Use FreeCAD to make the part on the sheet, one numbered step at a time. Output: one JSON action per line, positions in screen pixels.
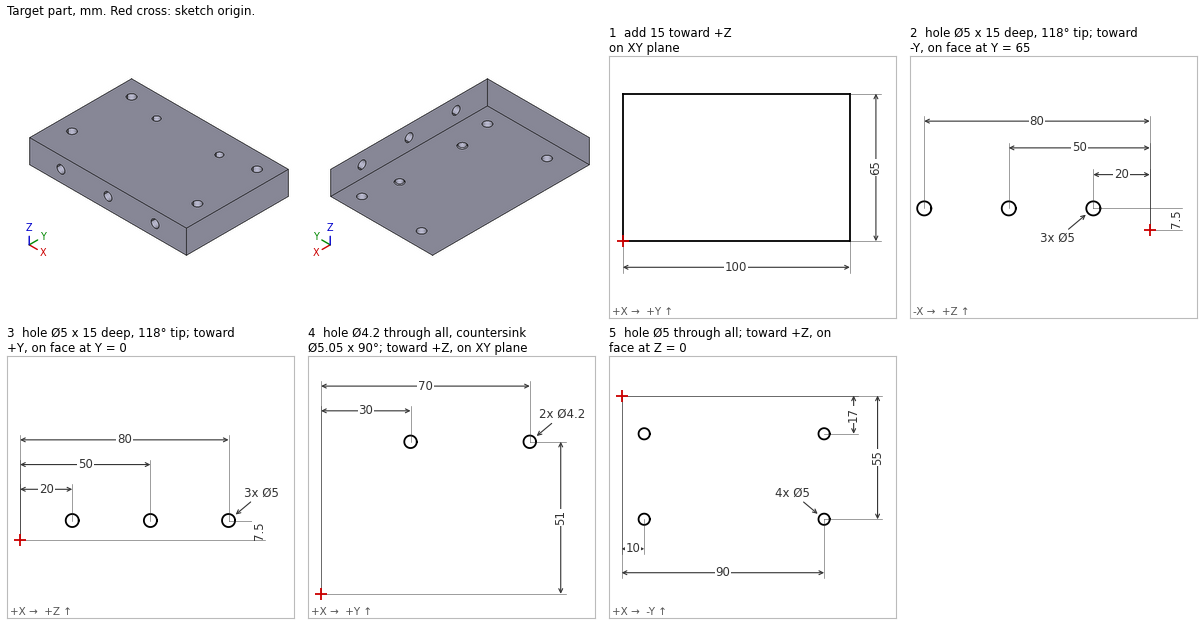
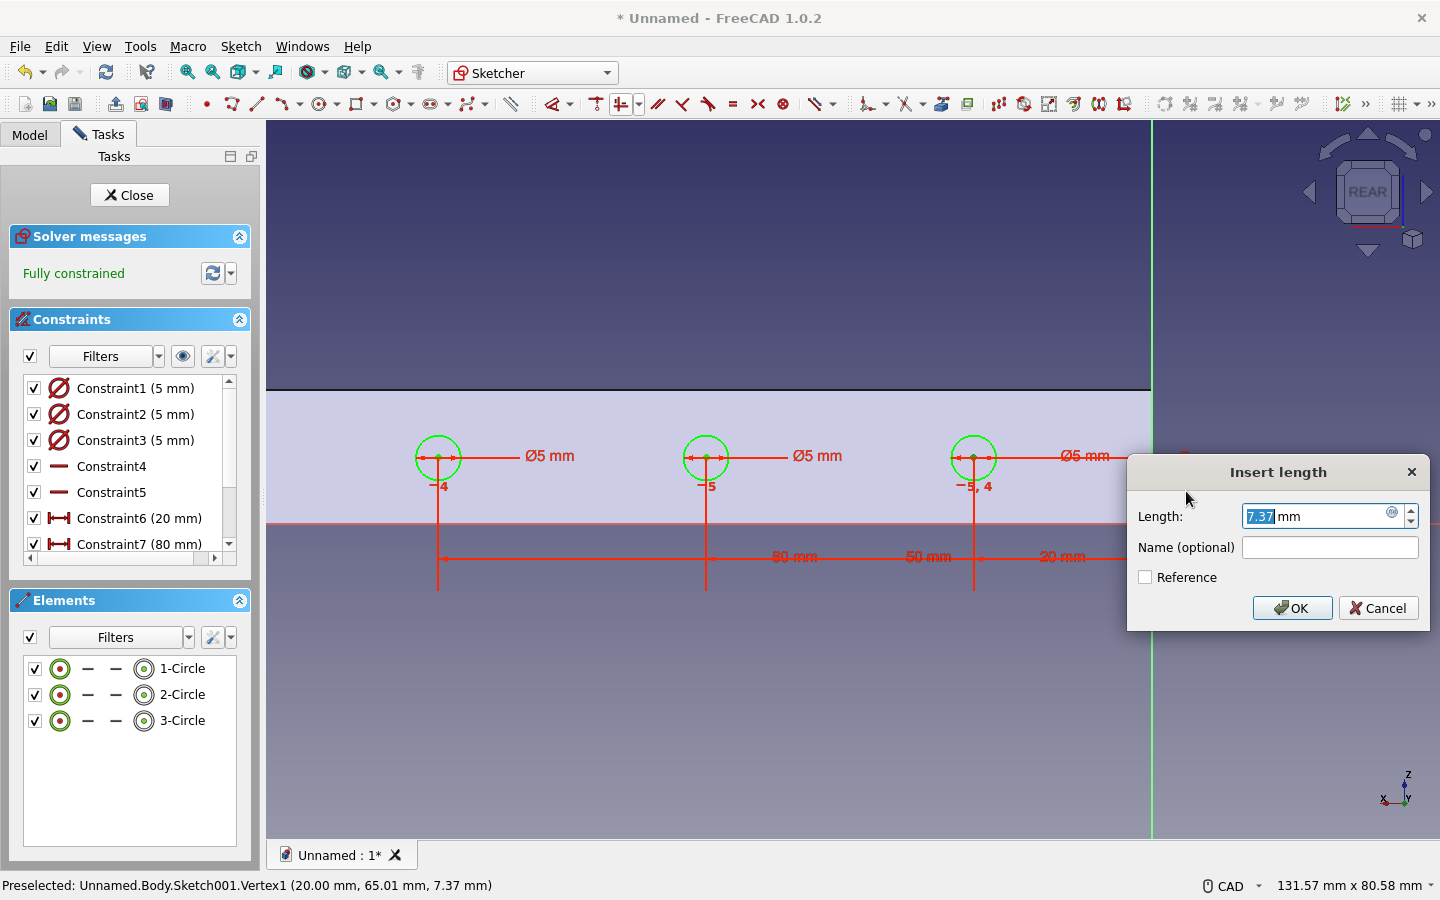
{"action": "type", "text": "7.5"}
{"action": "key", "text": "Return"}
{"action": "key", "text": "Escape"}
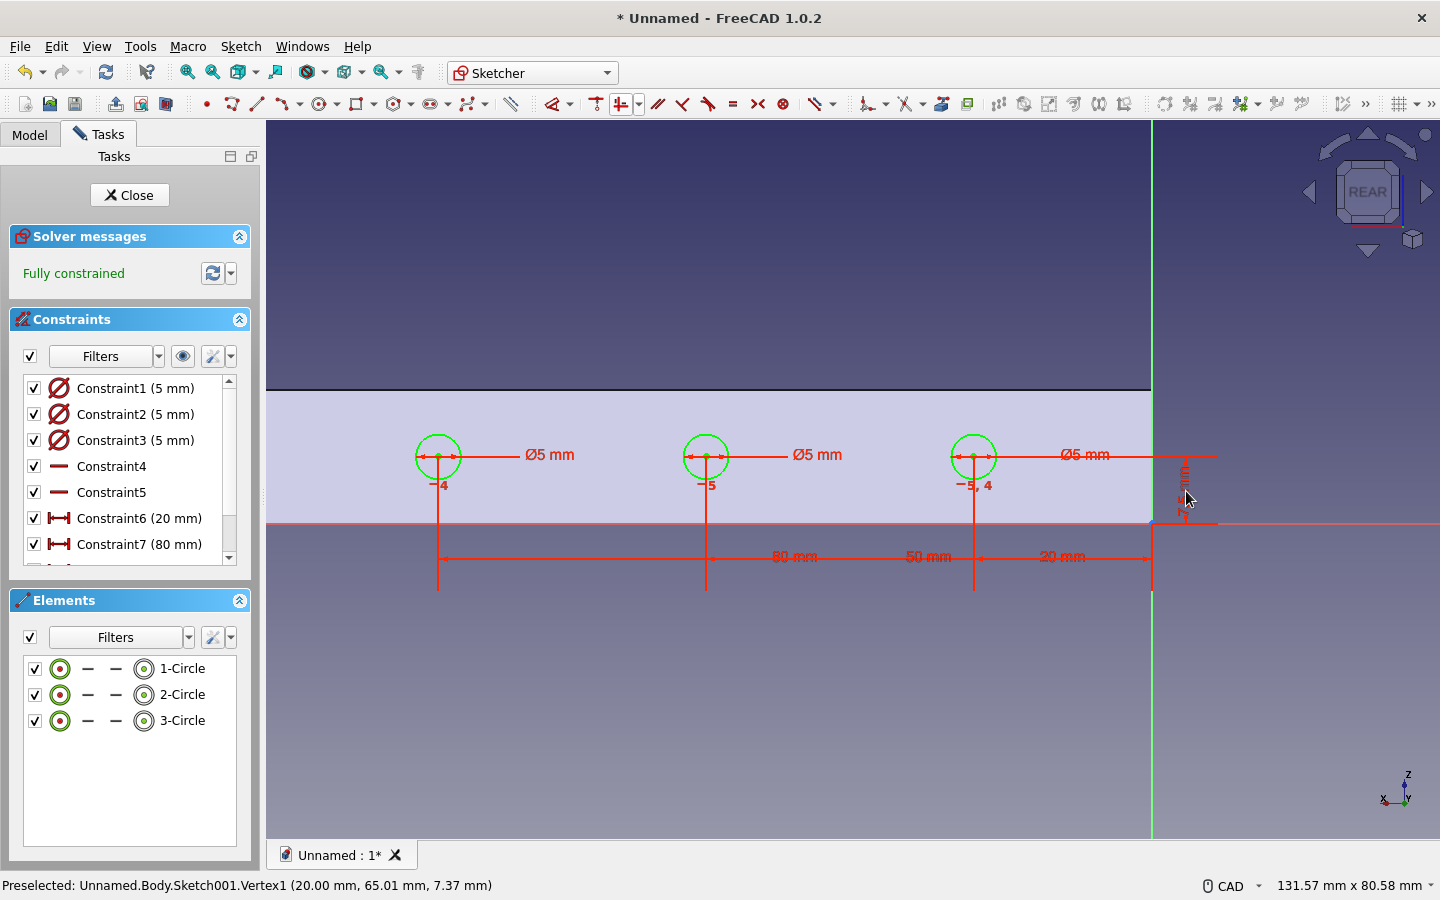
{"action": "left_click", "coordinate": [130, 195]}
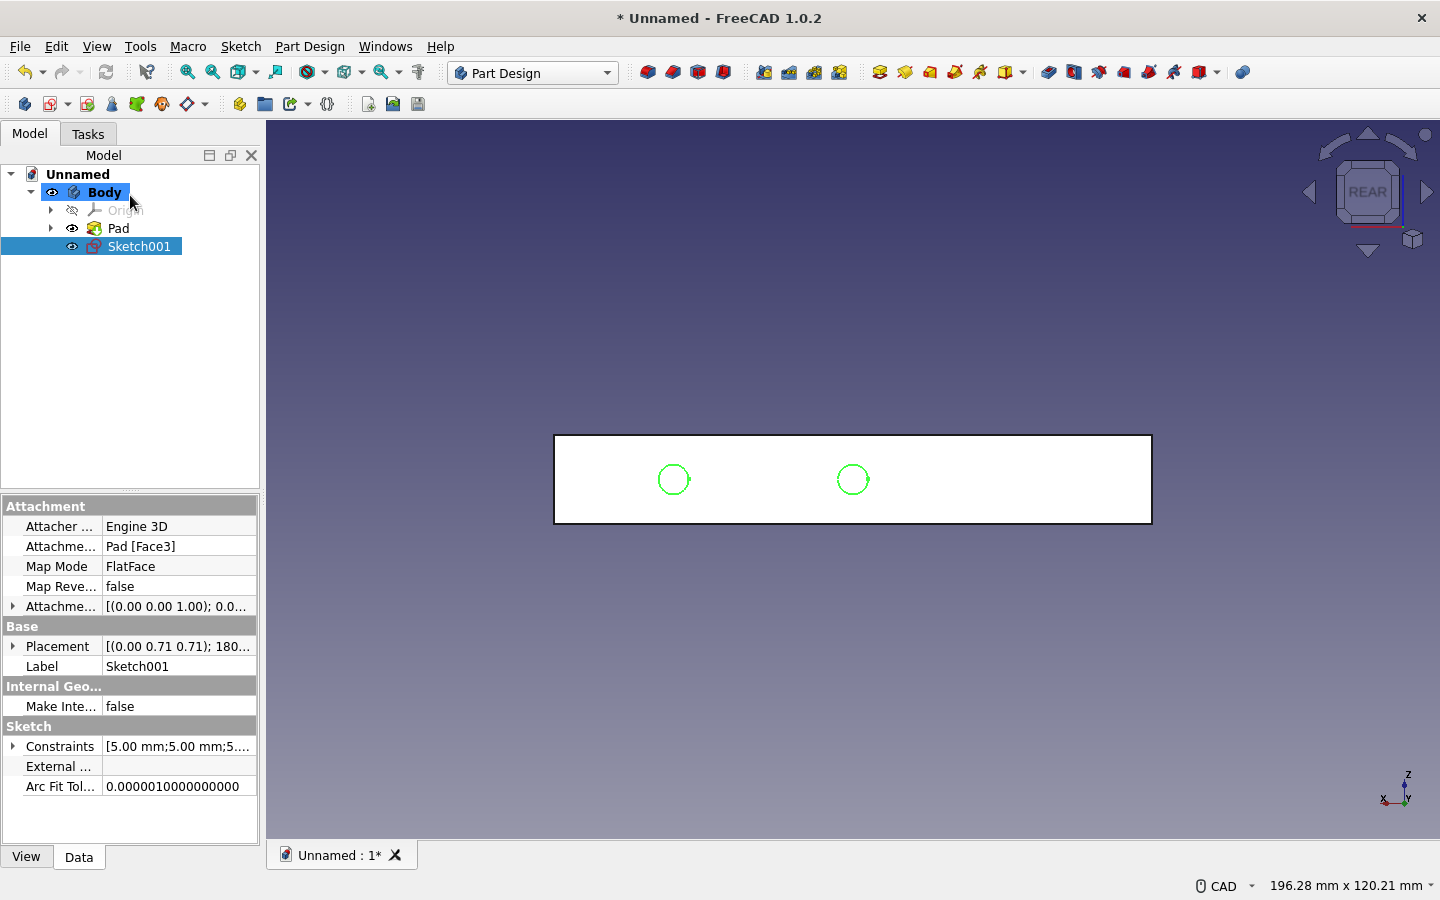
{"action": "left_click", "coordinate": [1074, 72]}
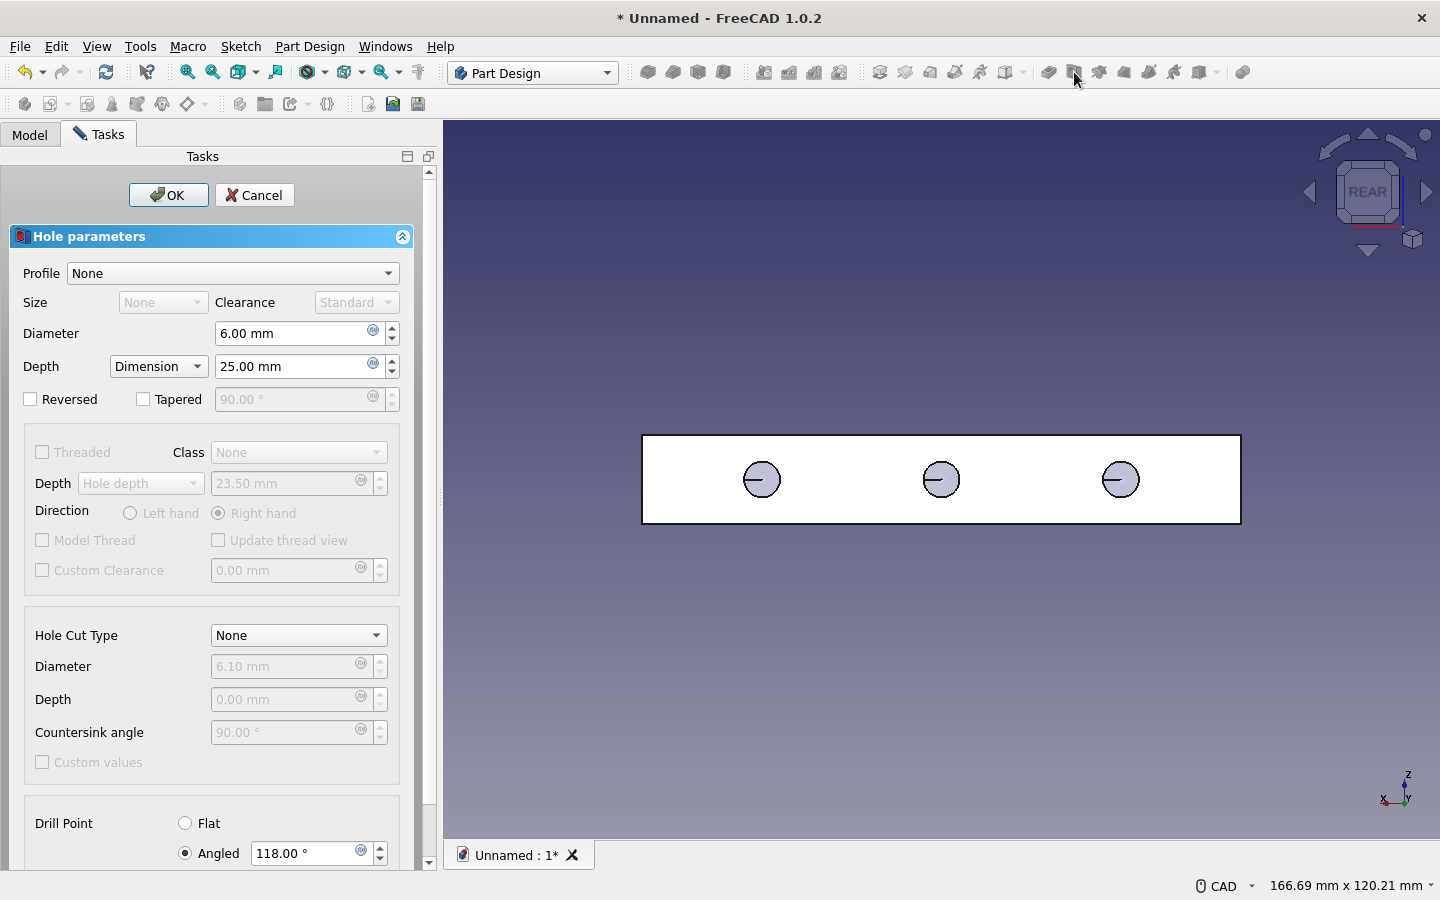
{"action": "triple_click", "coordinate": [300, 334]}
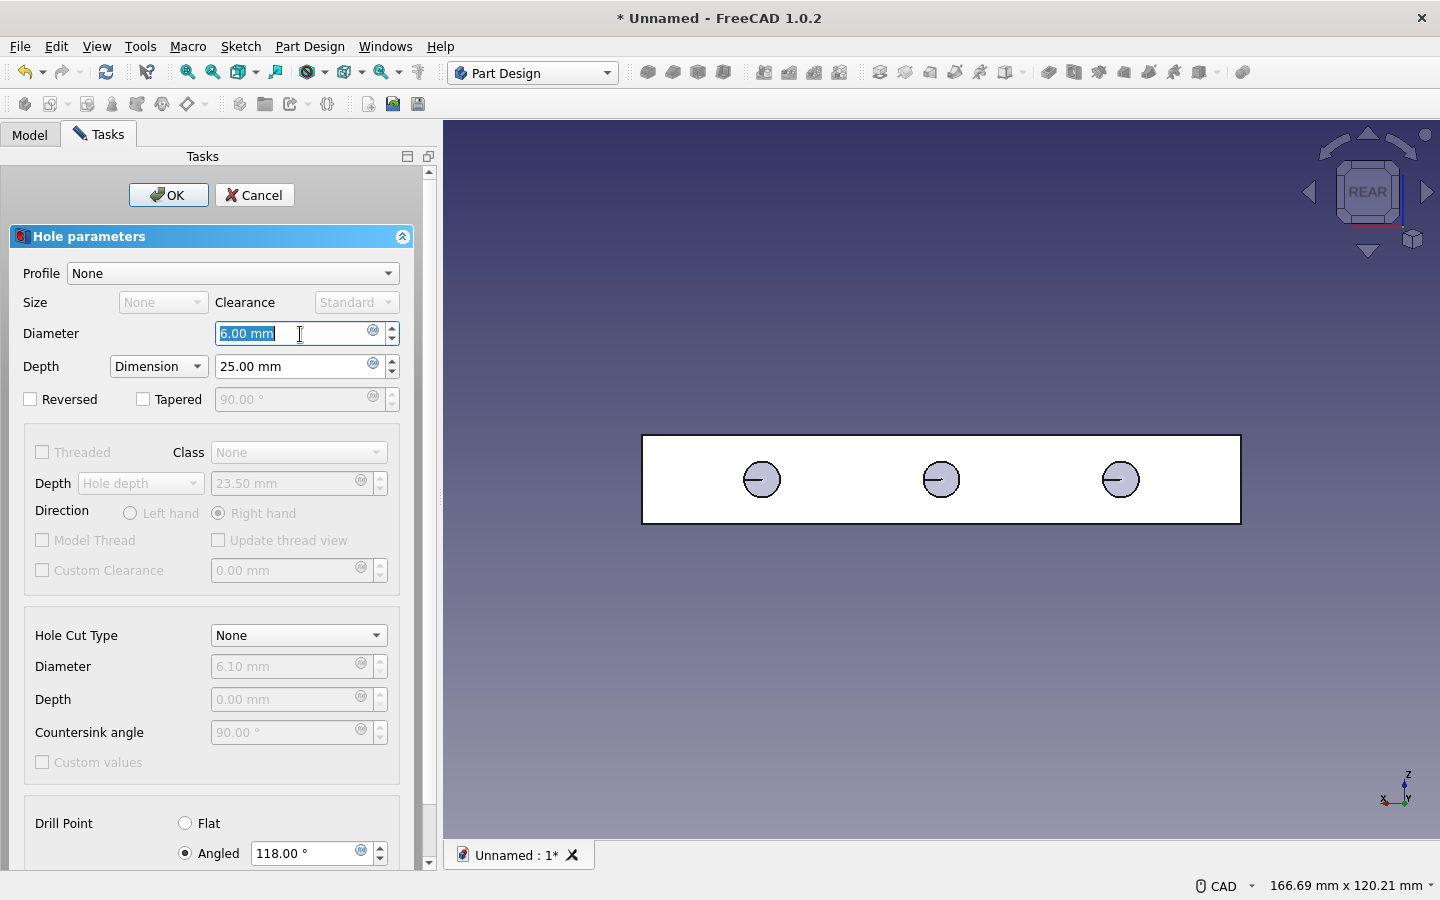
{"action": "type", "text": "5"}
{"action": "key", "text": "Tab"}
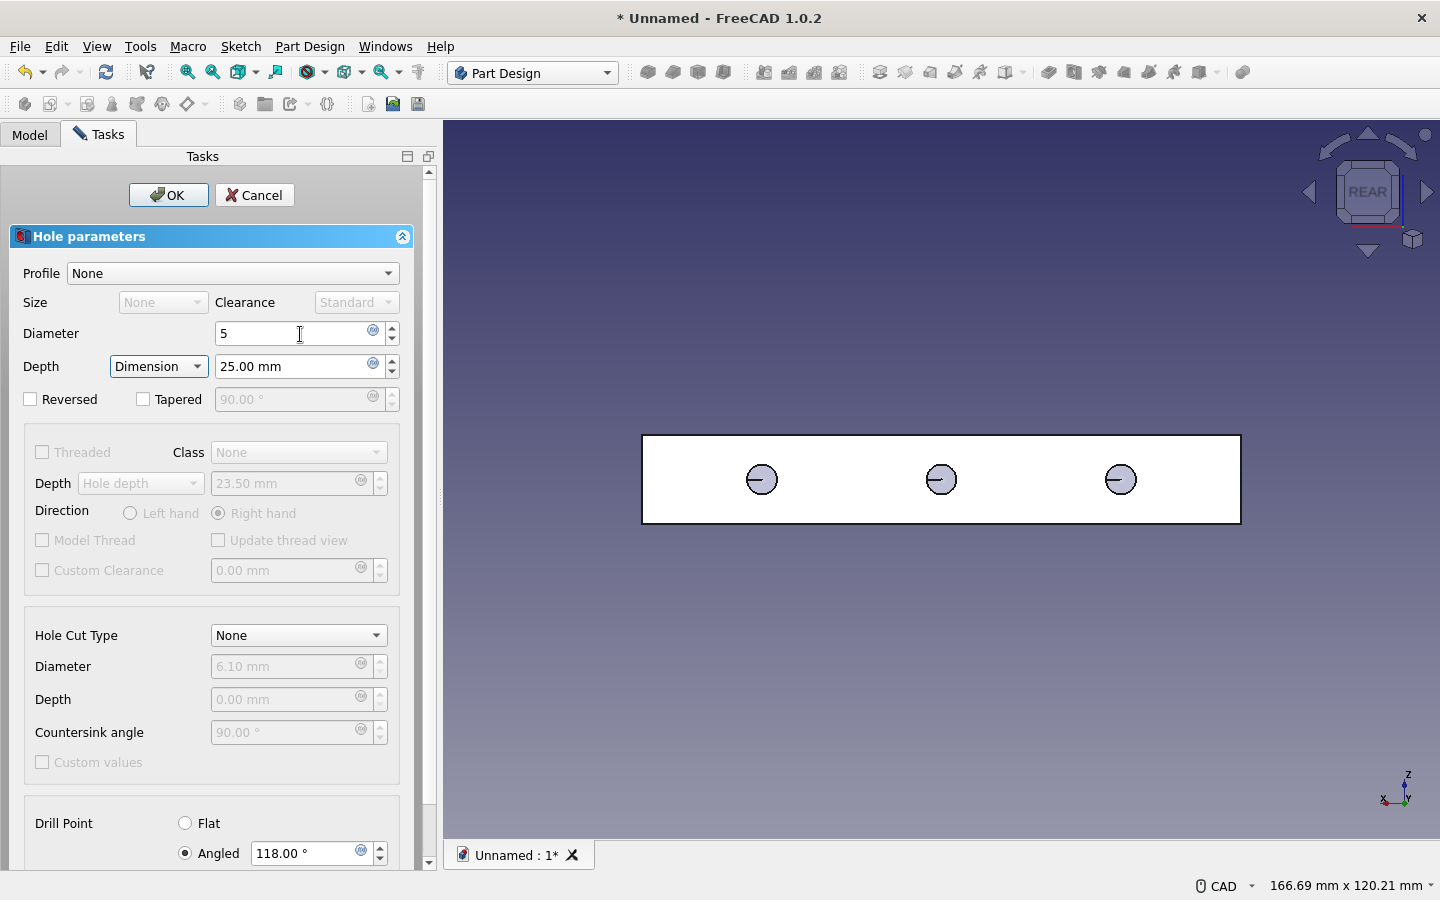
{"action": "triple_click", "coordinate": [300, 366]}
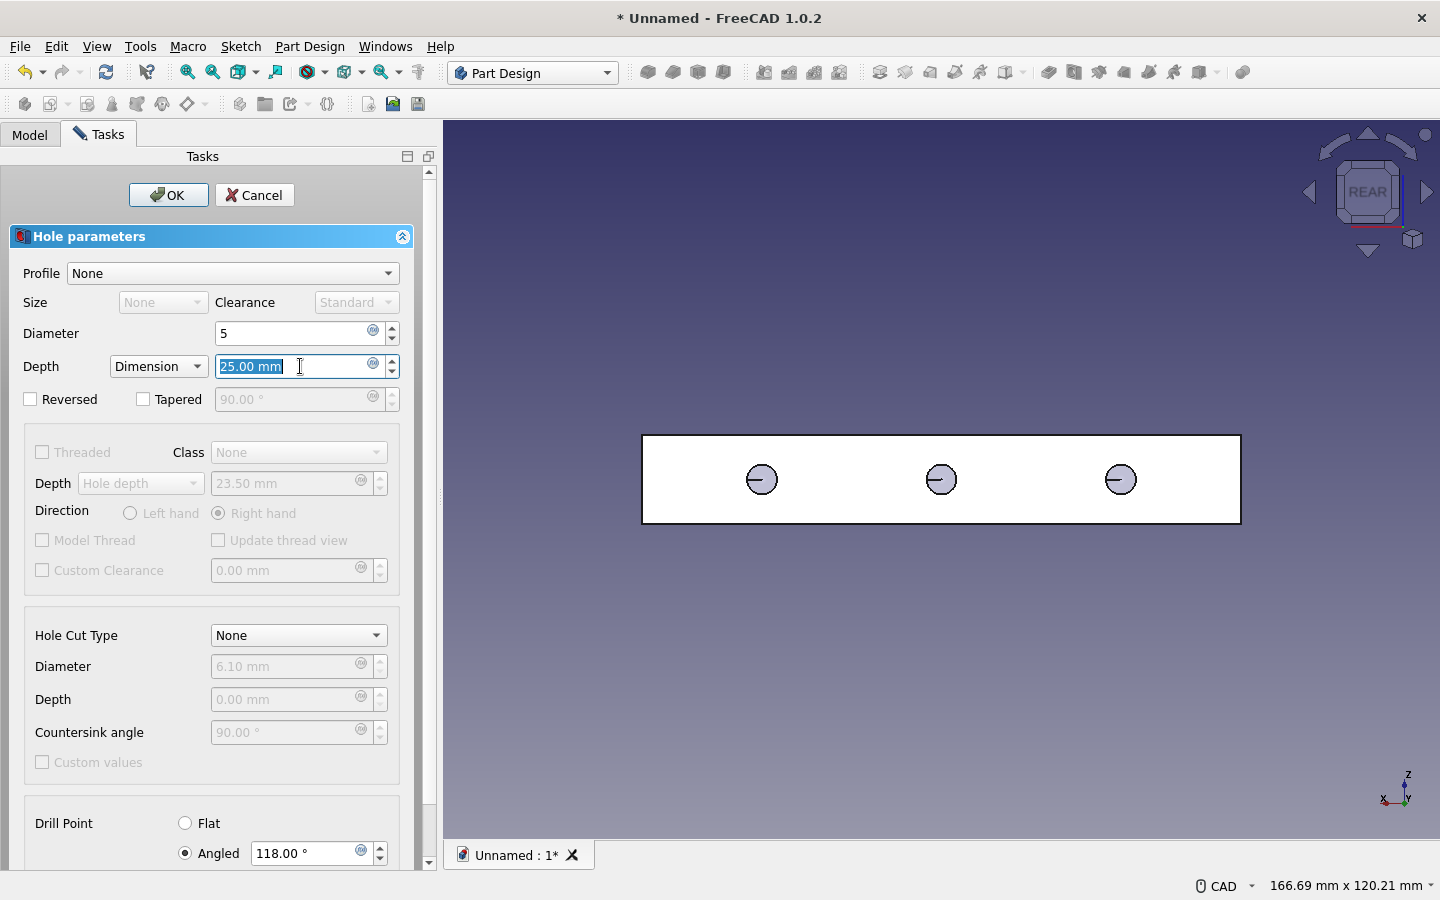
{"action": "type", "text": "15"}
{"action": "key", "text": "Tab"}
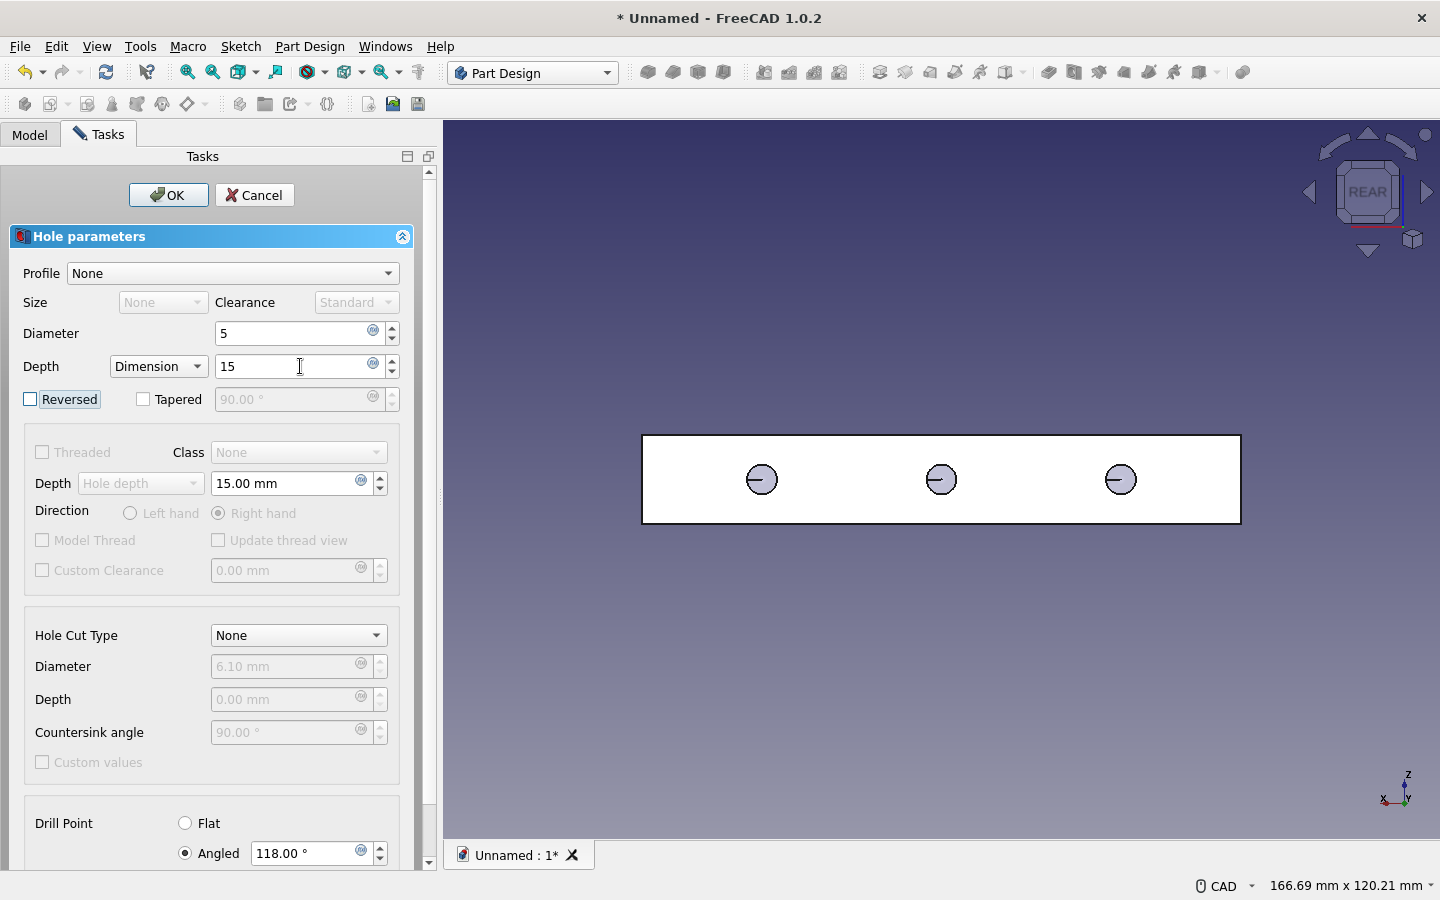
{"action": "left_click", "coordinate": [169, 195]}